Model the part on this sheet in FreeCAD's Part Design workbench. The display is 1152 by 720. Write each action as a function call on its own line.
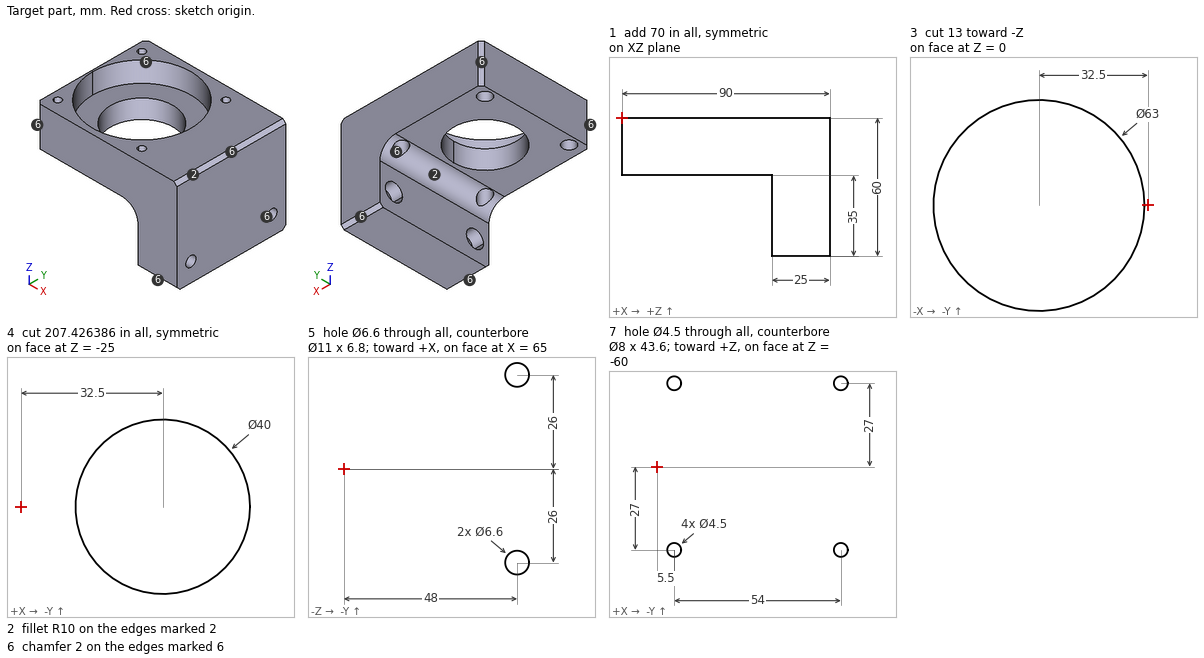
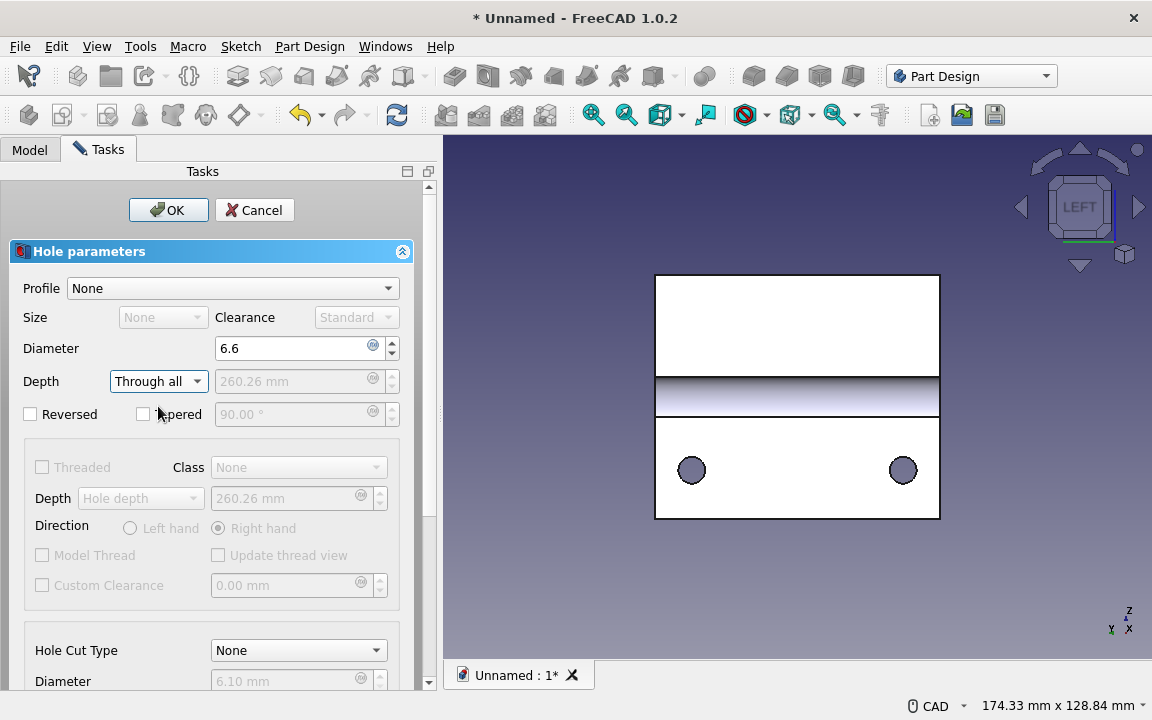
click(300, 650)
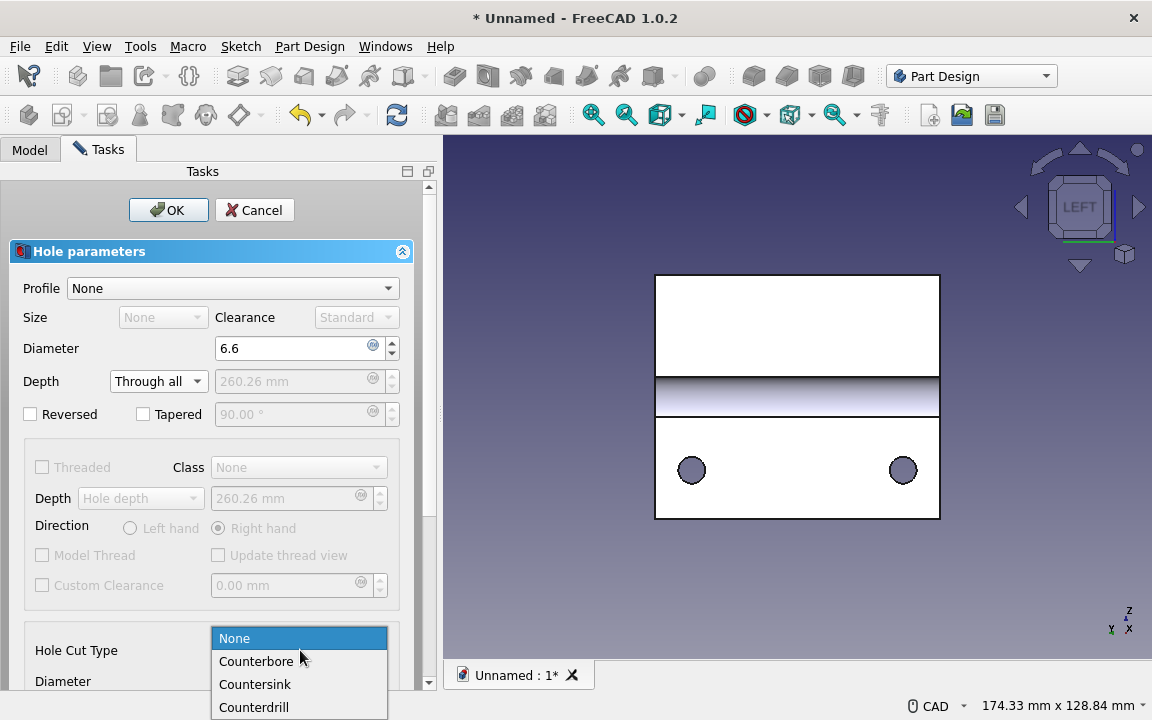
click(298, 662)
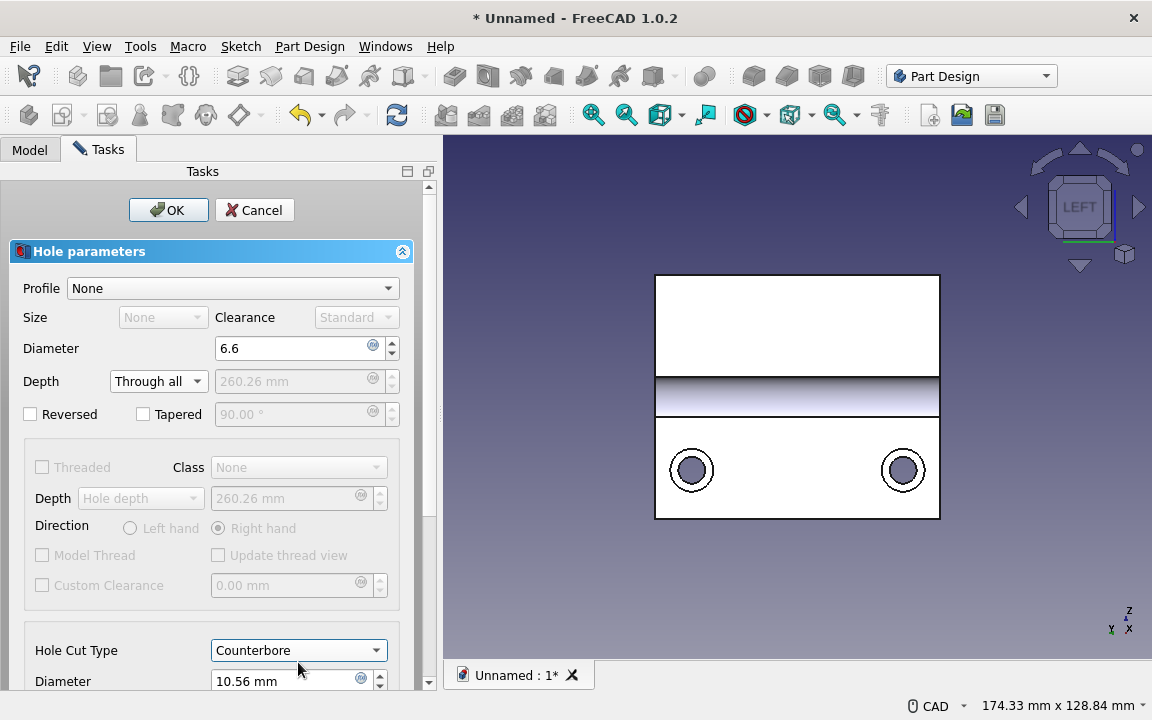
scroll(429, 436, down, 2)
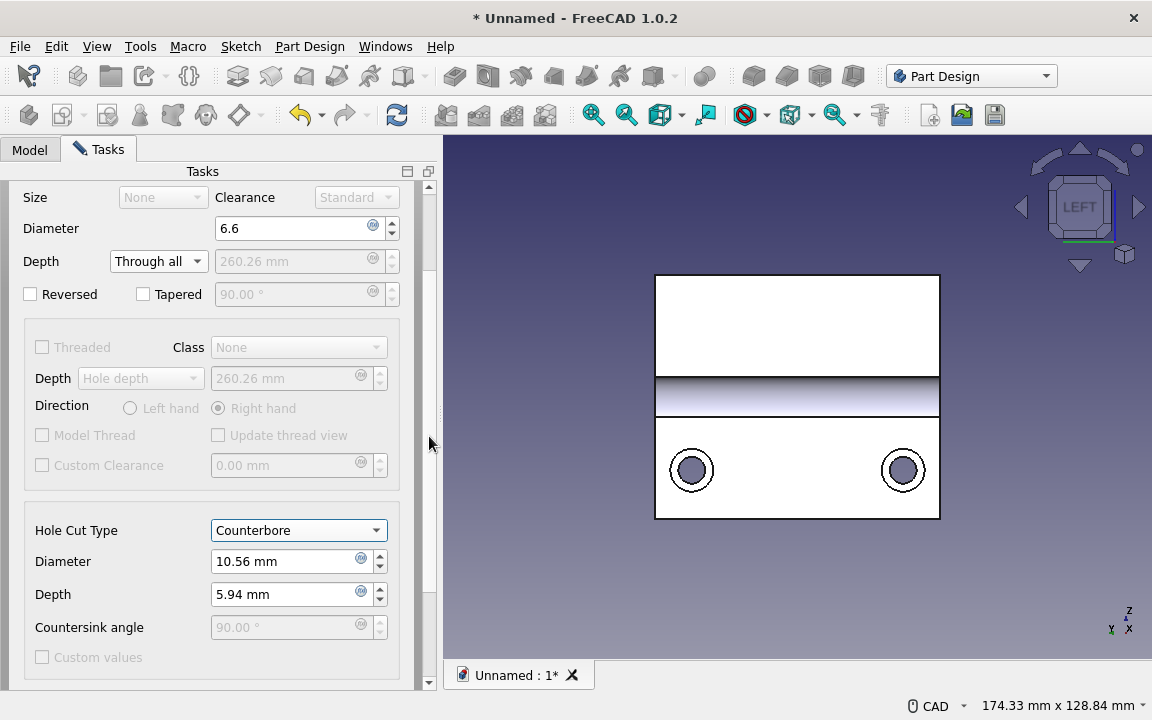
triple_click(292, 562)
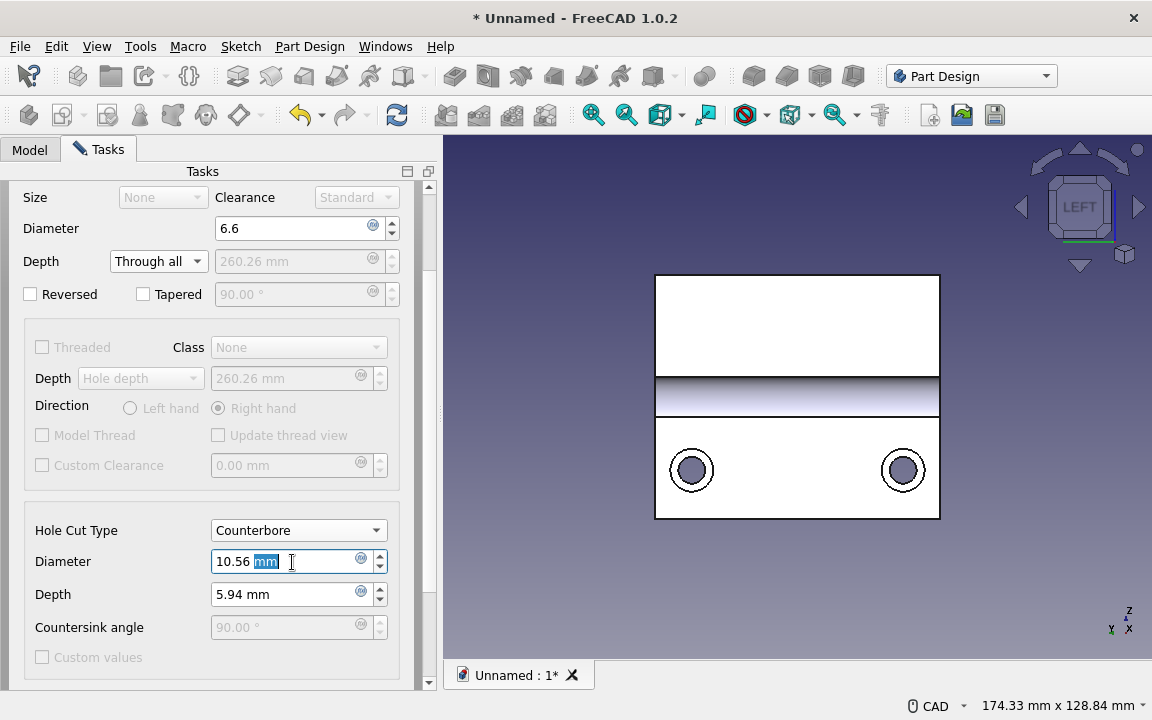
text(11)
key(Tab)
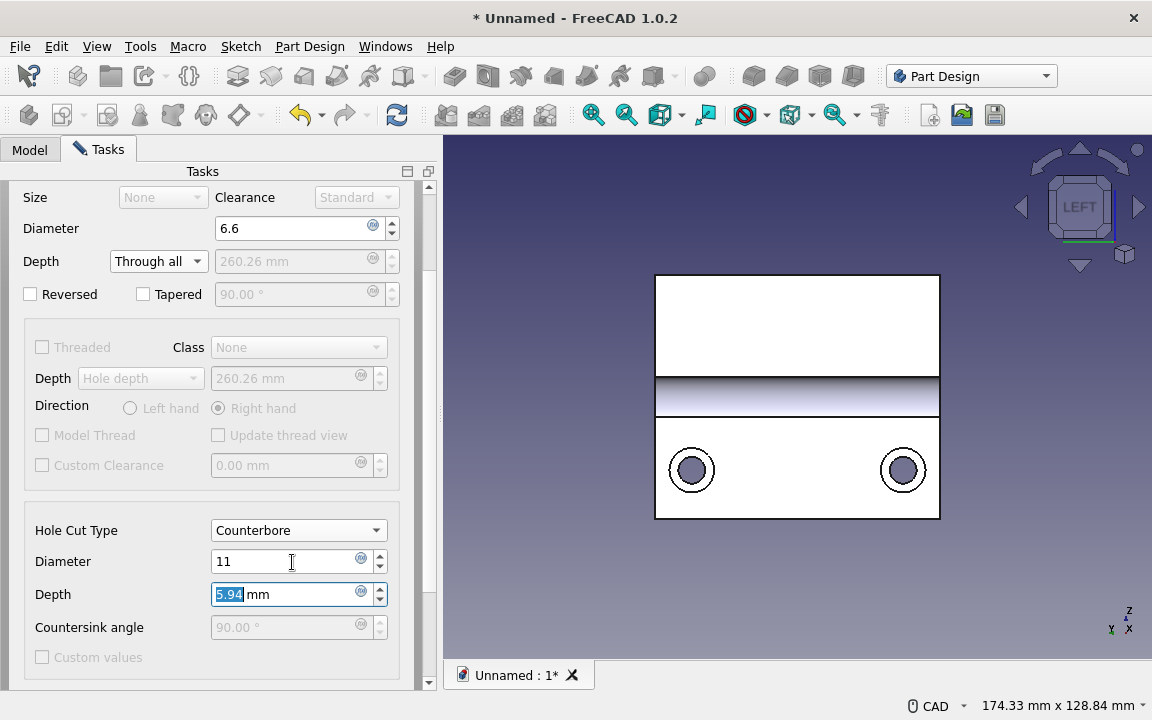
text(6.8)
key(Tab)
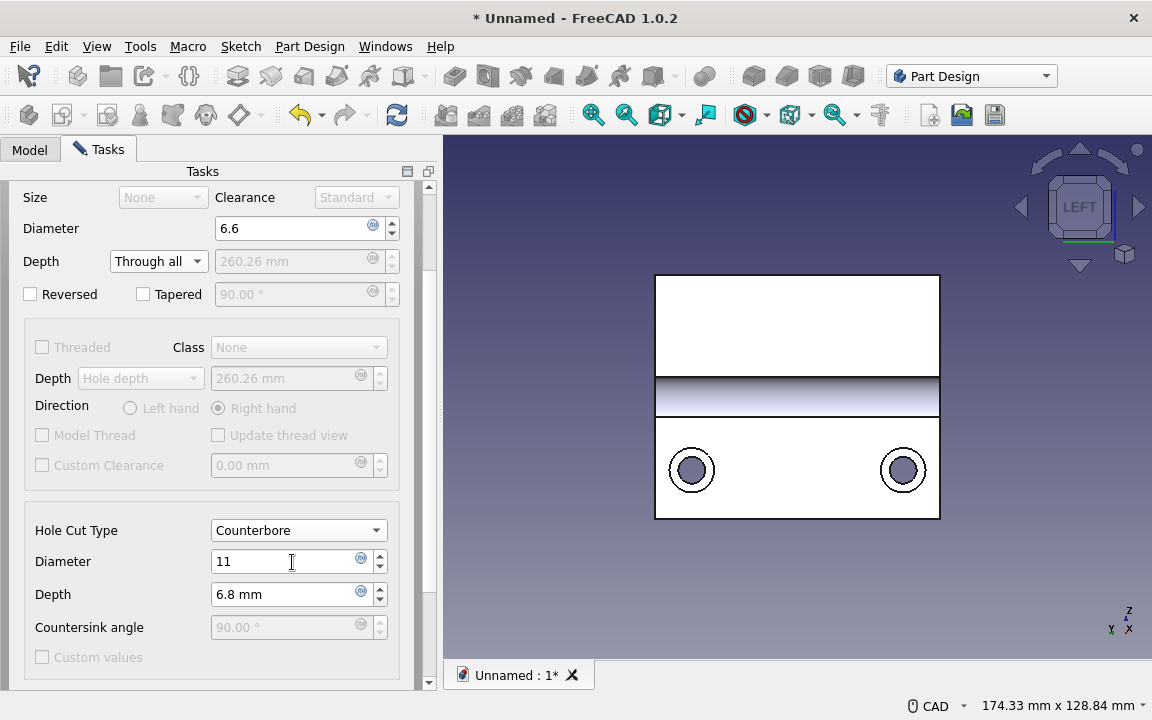
scroll(429, 436, up, 3)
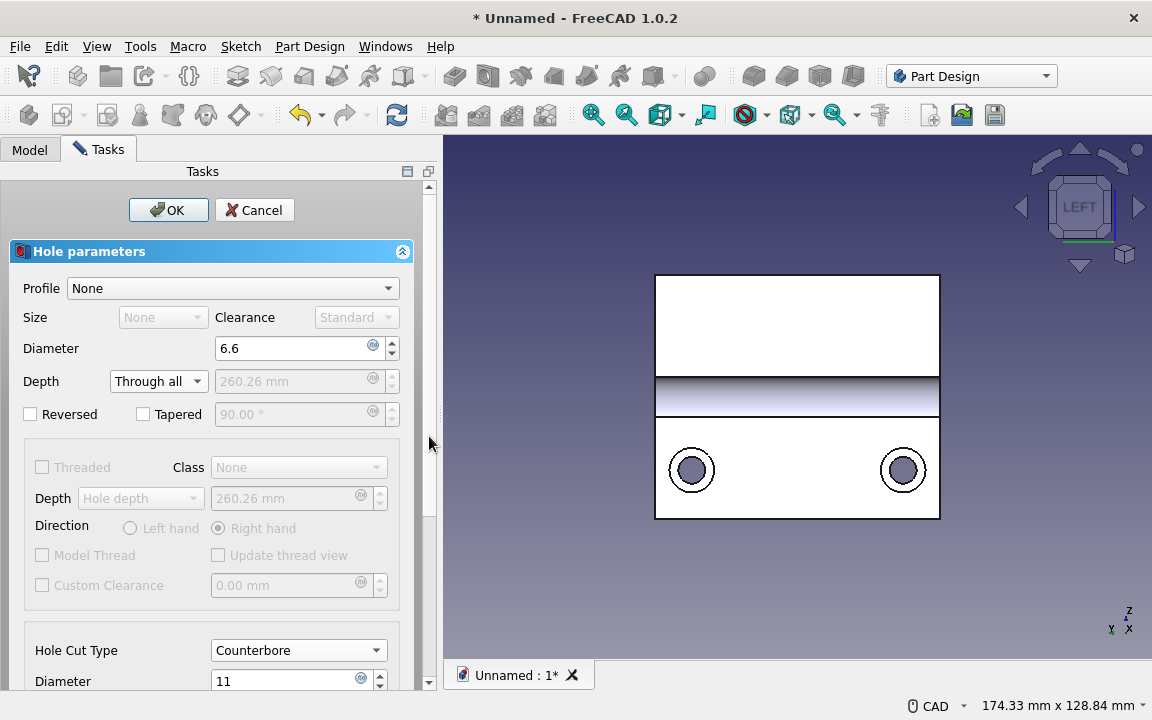
click(169, 210)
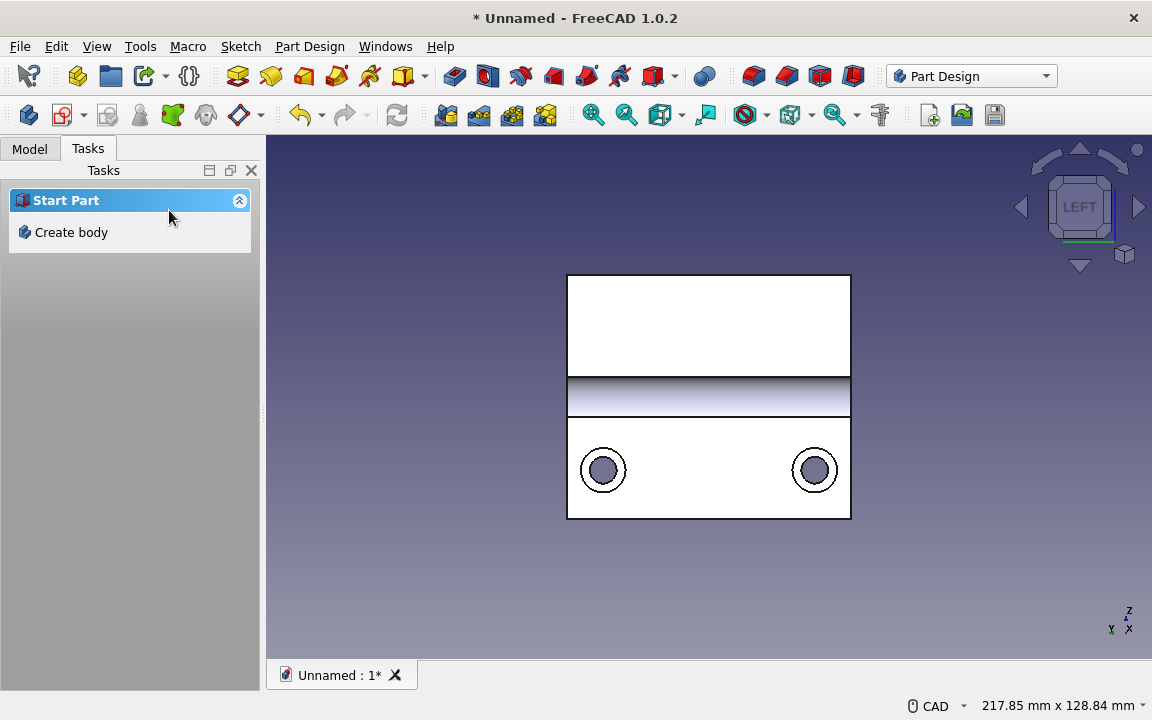
click(851, 325)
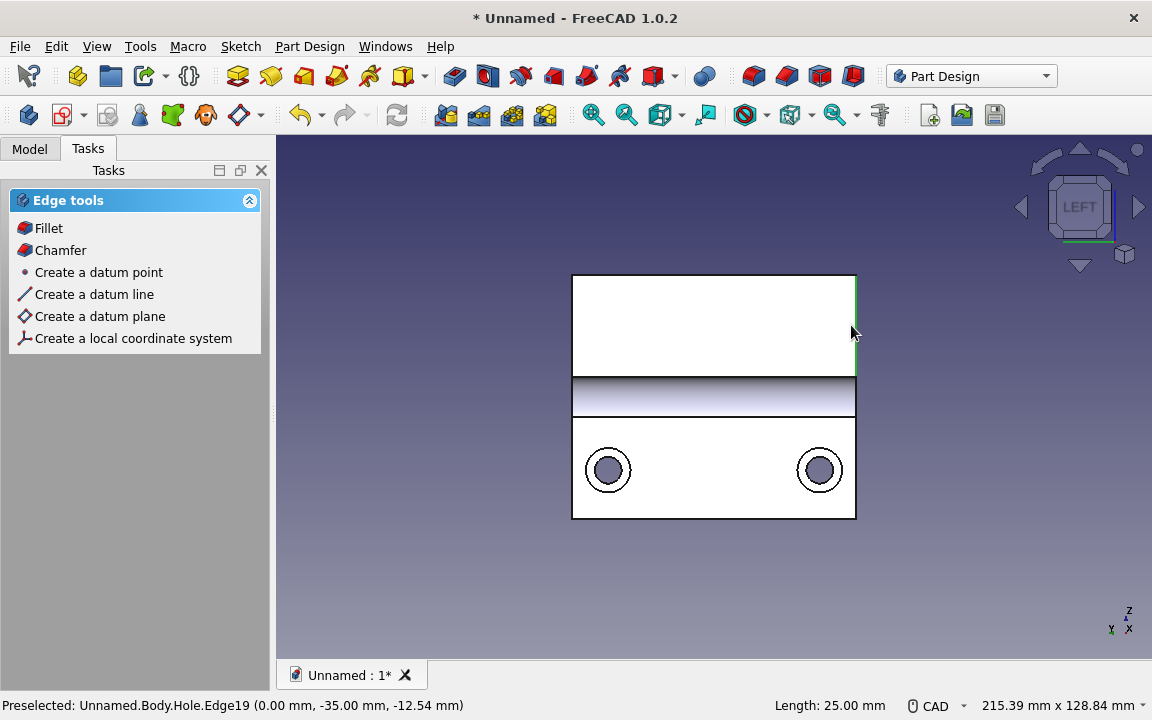
key(0)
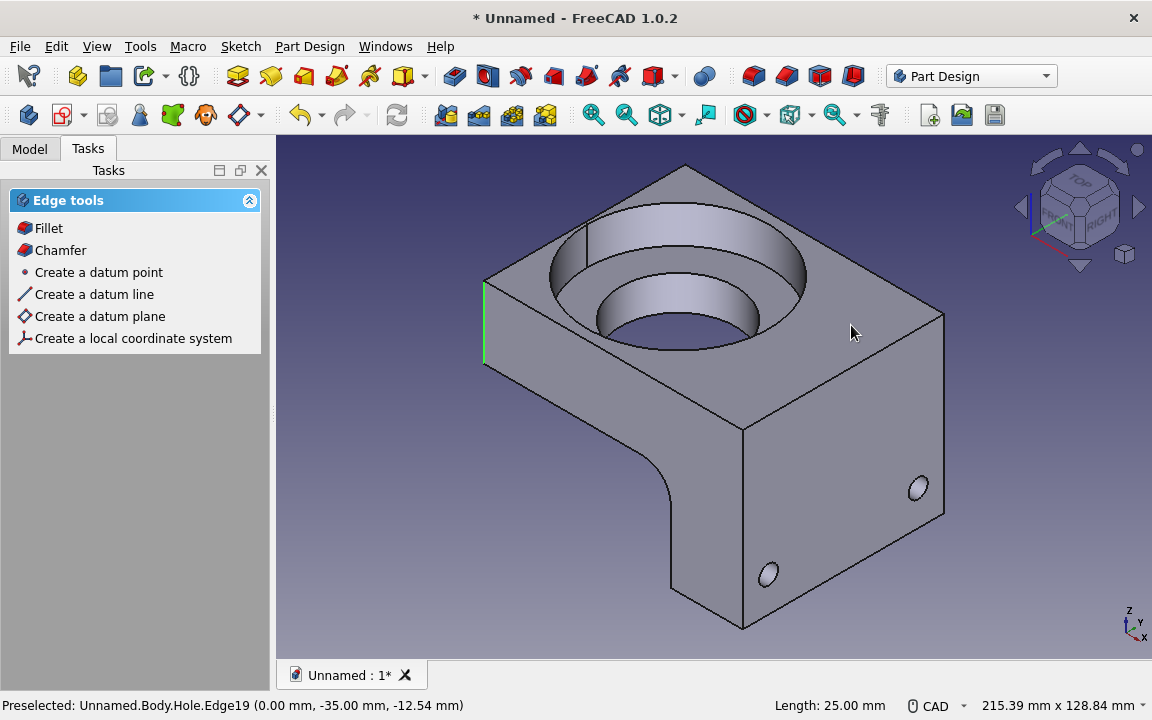
click(843, 371, ctrl)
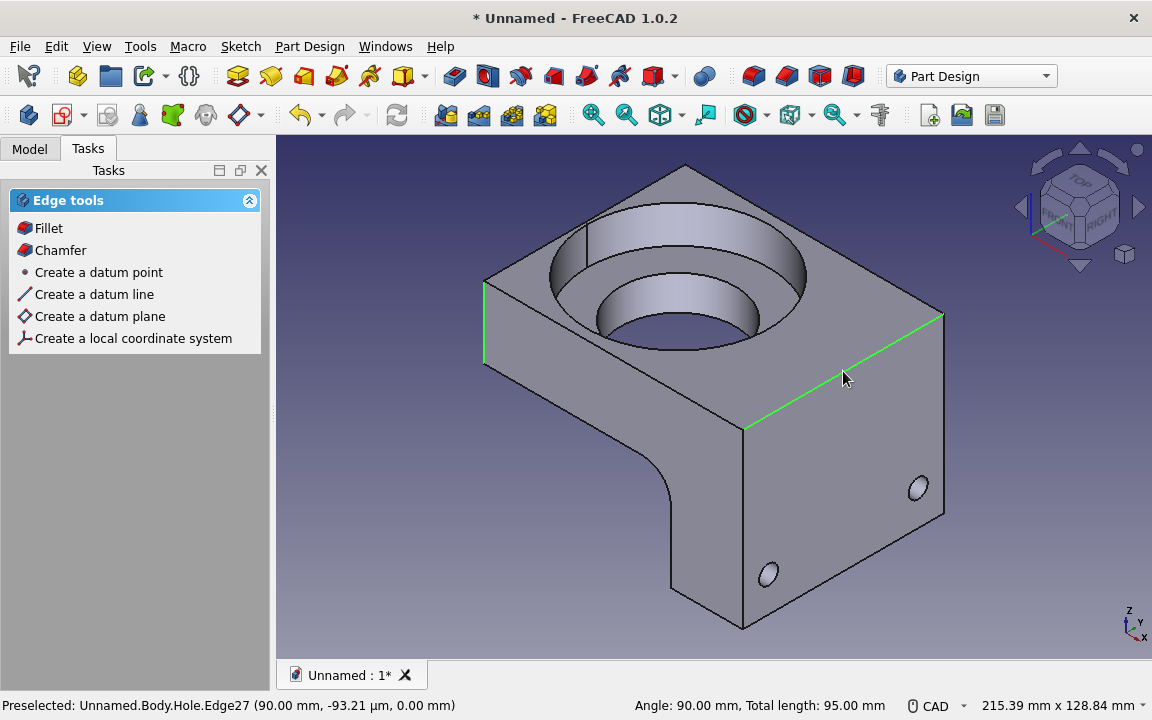
key(2)